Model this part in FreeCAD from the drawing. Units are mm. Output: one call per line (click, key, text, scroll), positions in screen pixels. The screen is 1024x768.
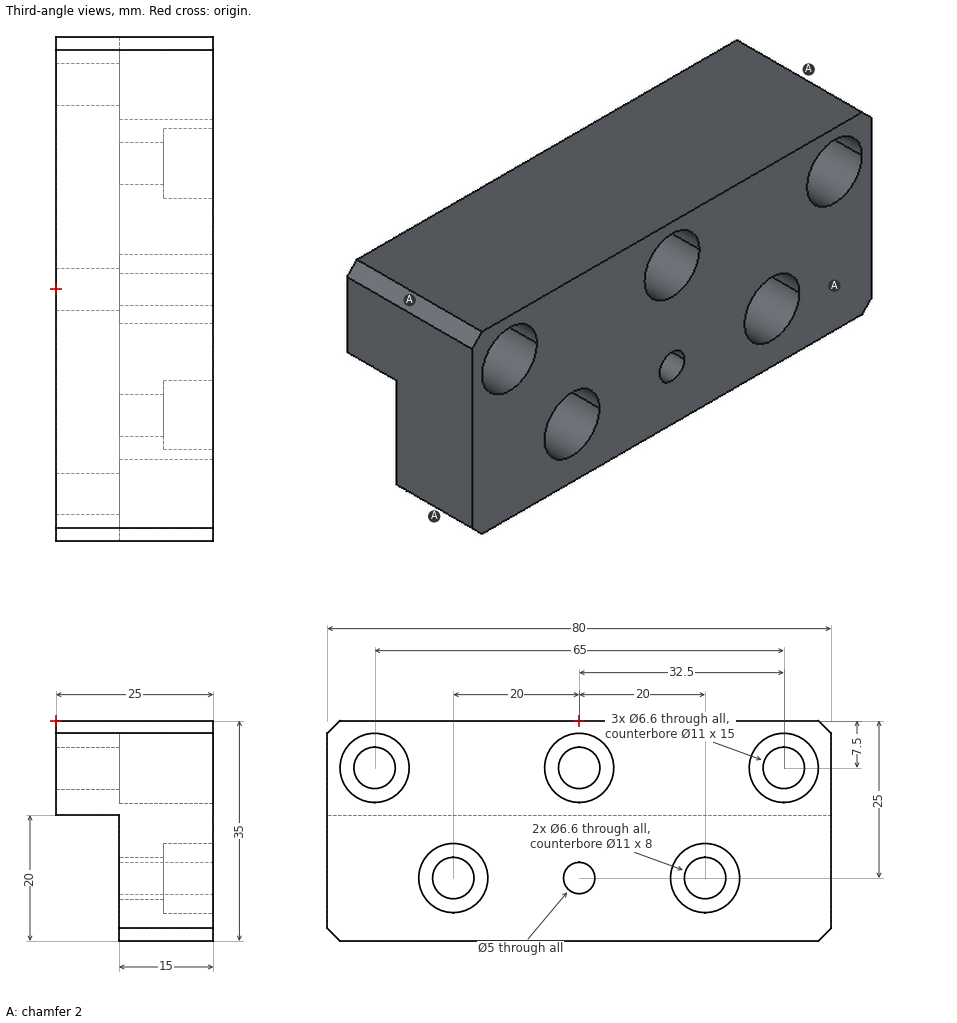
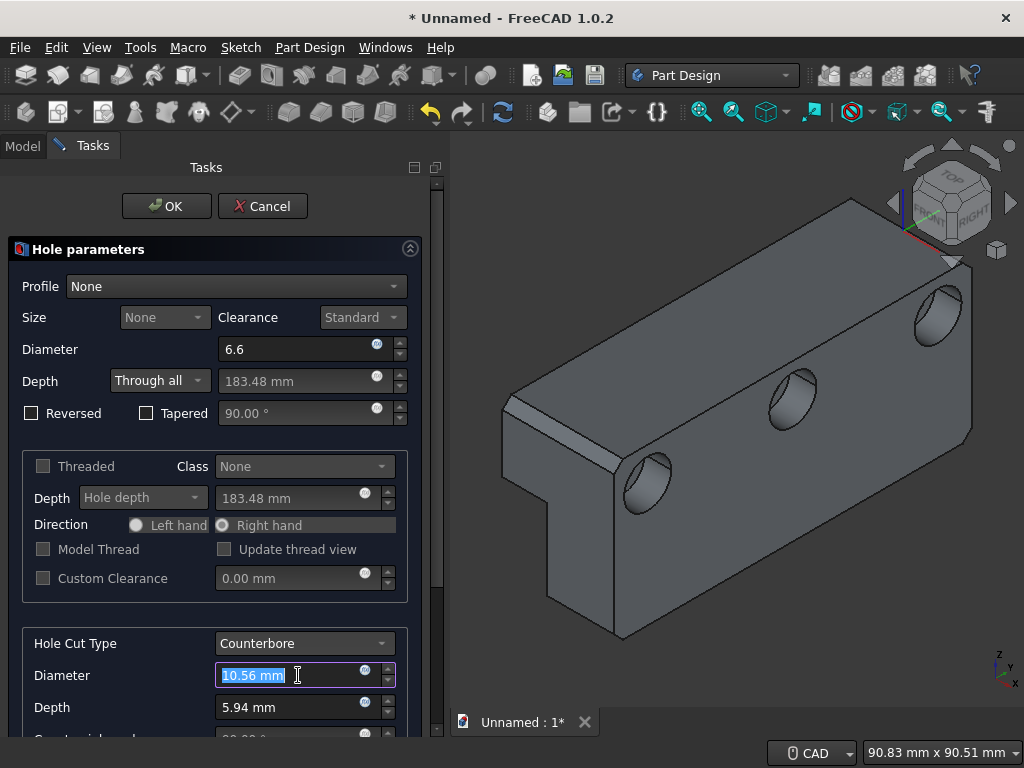
text(11)
key(Tab)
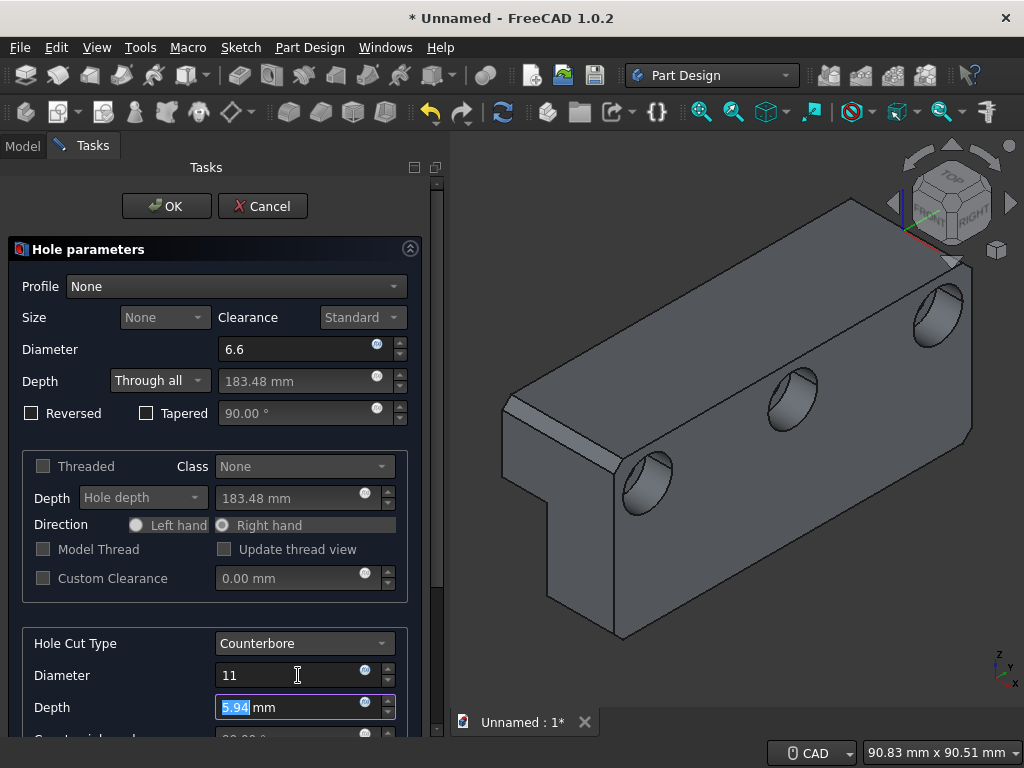
text(15)
key(Tab)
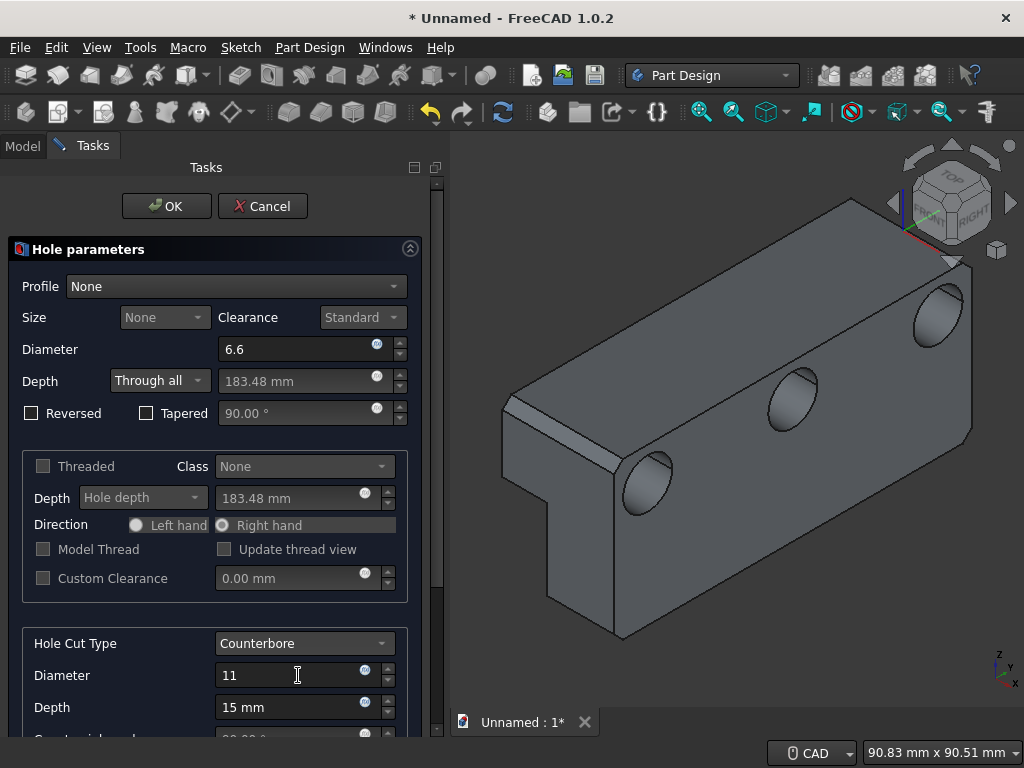
click(167, 206)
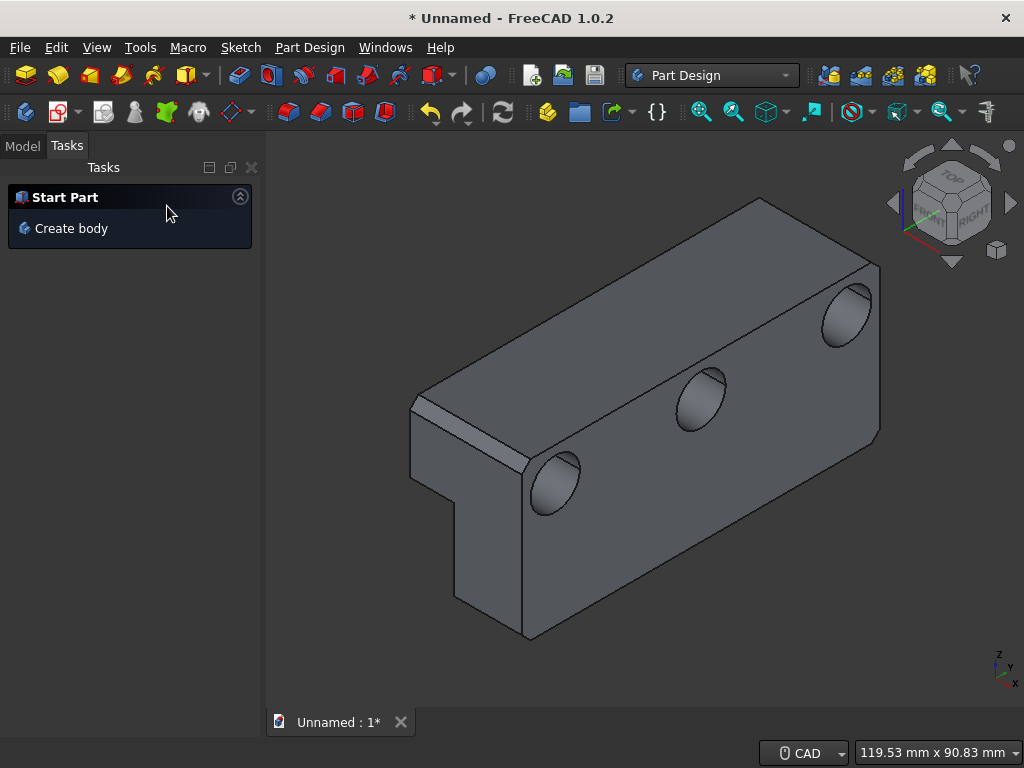
click(752, 447)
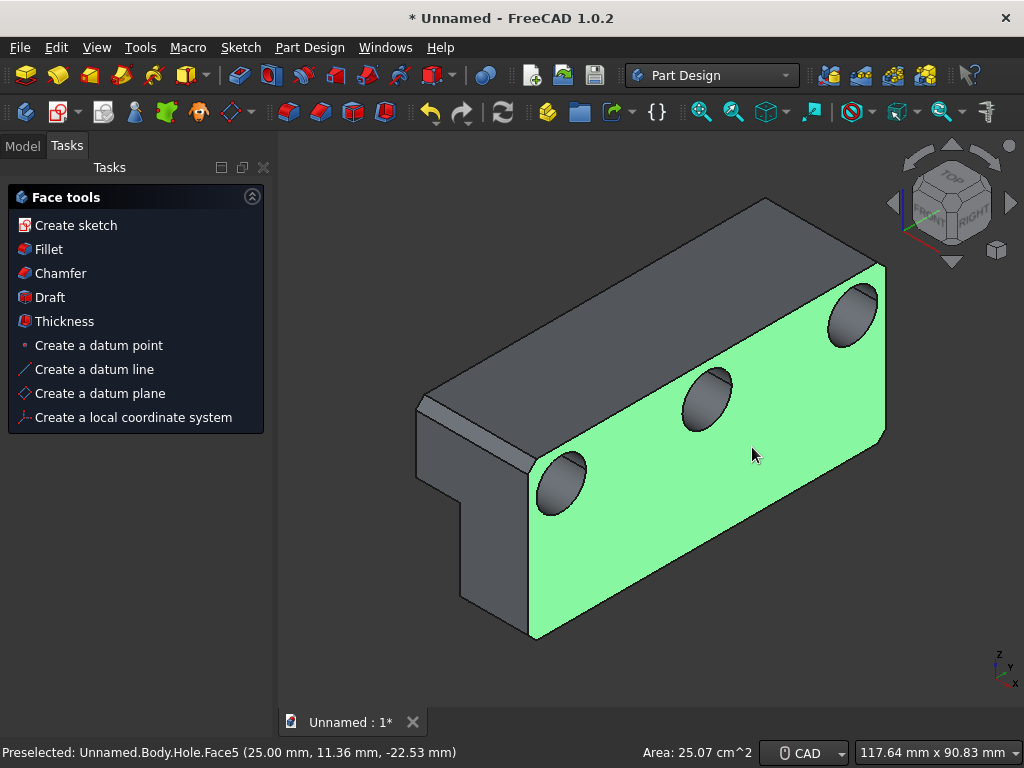
click(58, 112)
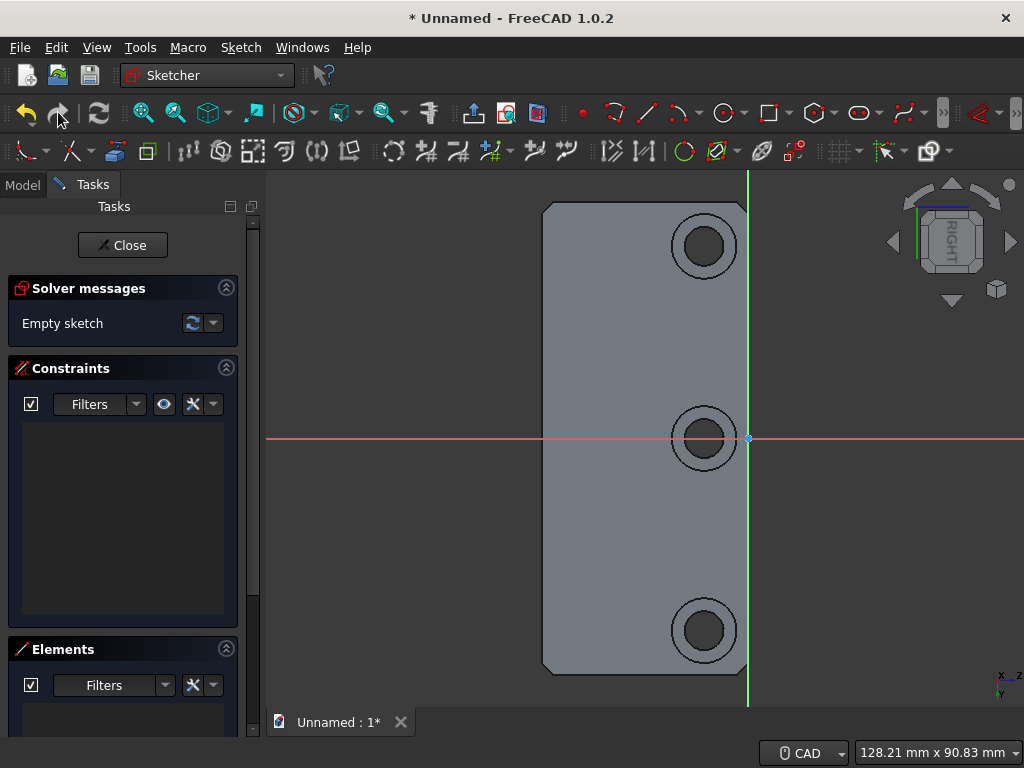
scroll(603, 438, up, 12)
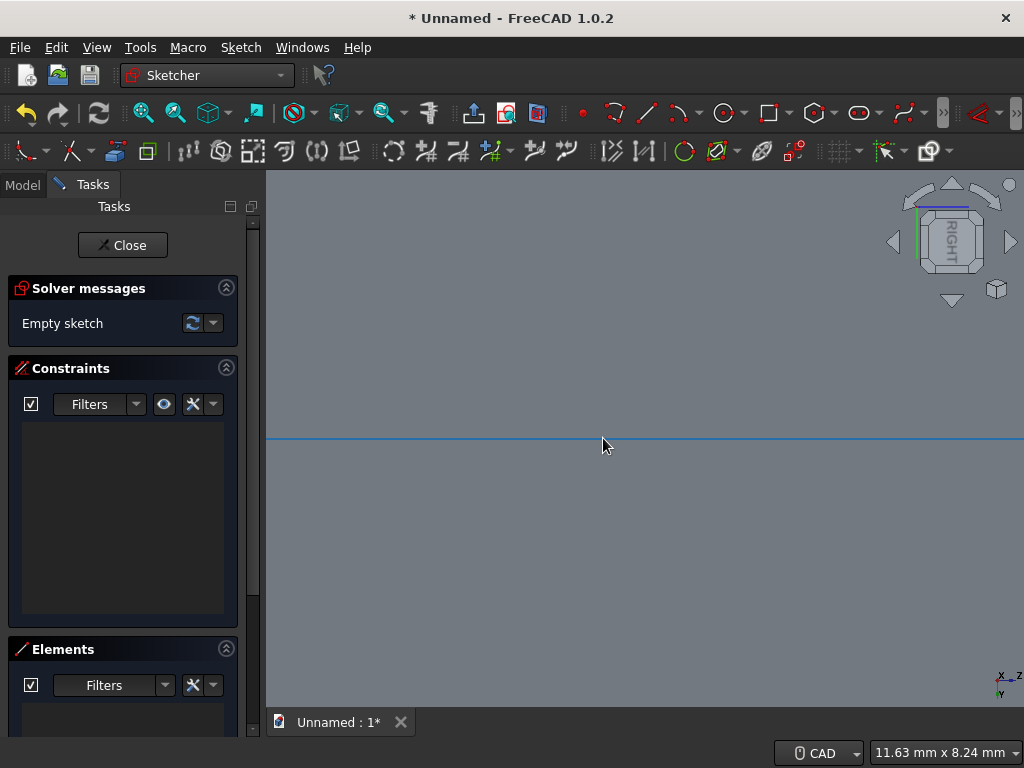
click(724, 114)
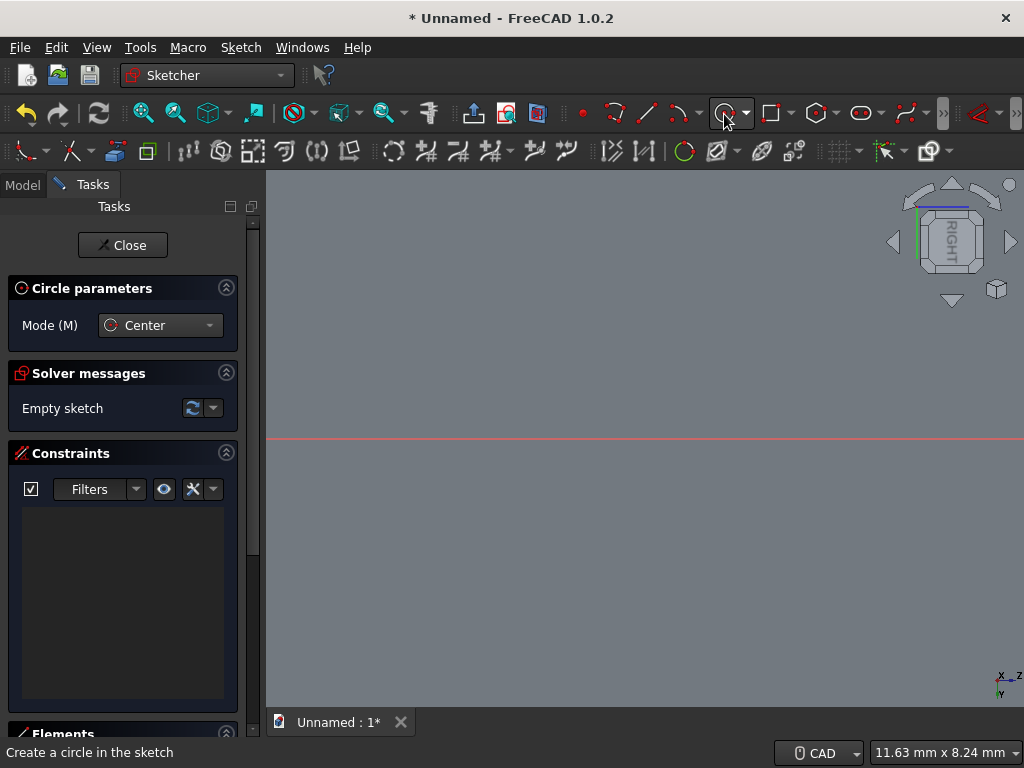
click(573, 438)
click(688, 323)
key(Escape)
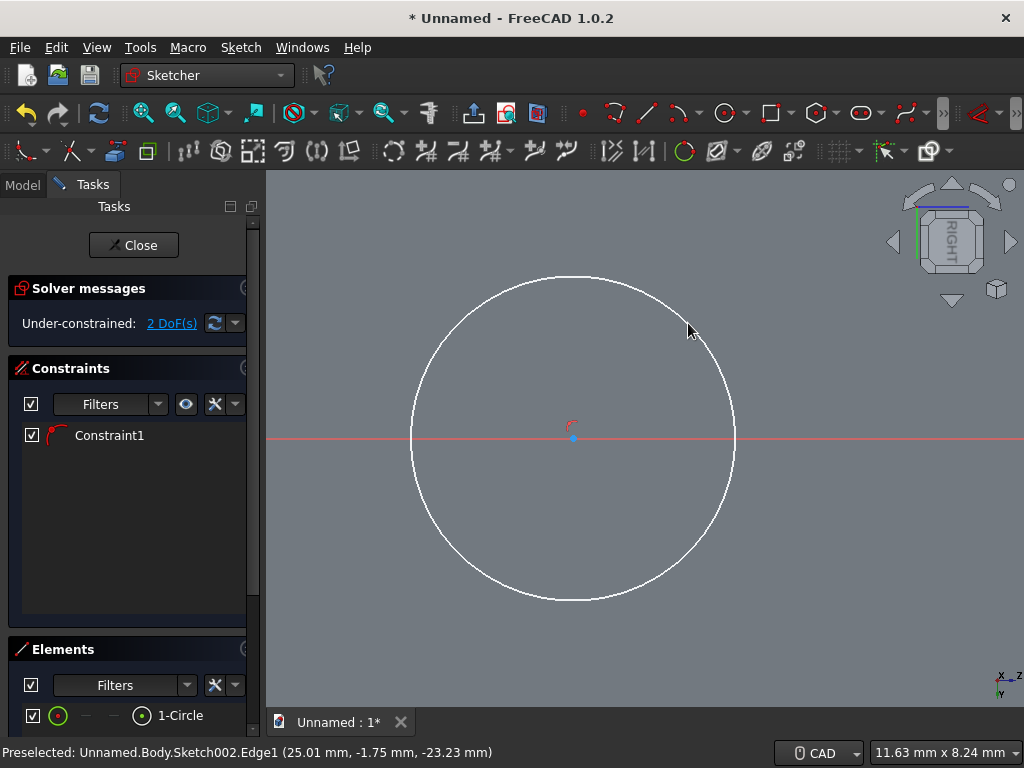
click(978, 114)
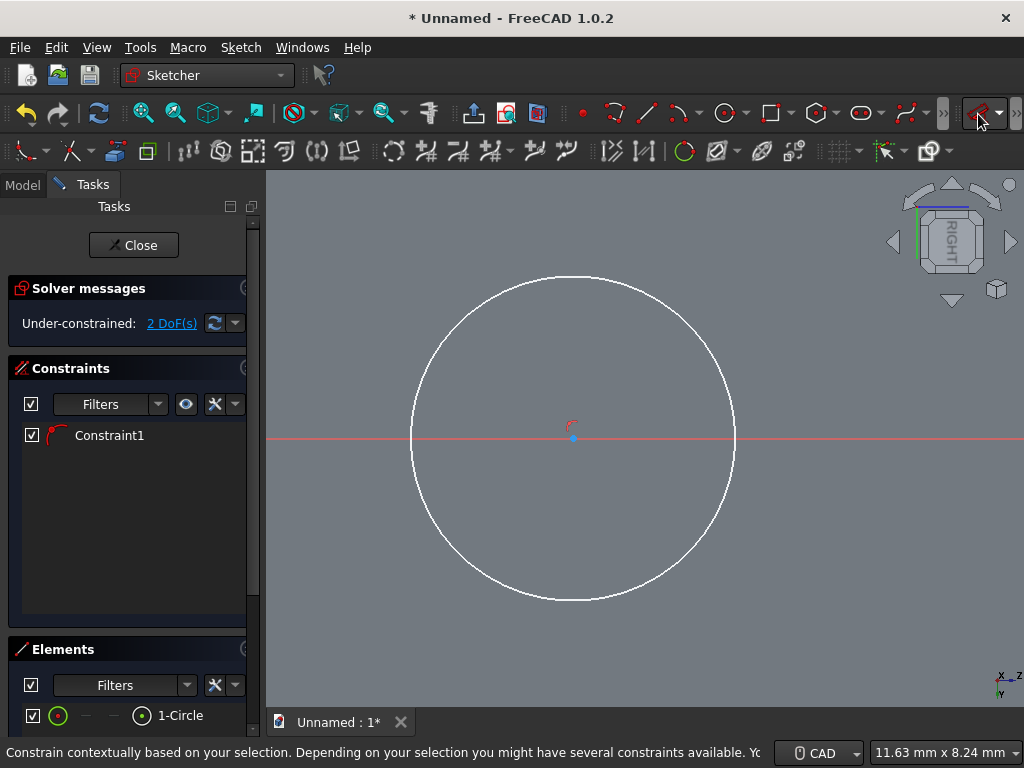
click(687, 323)
click(709, 300)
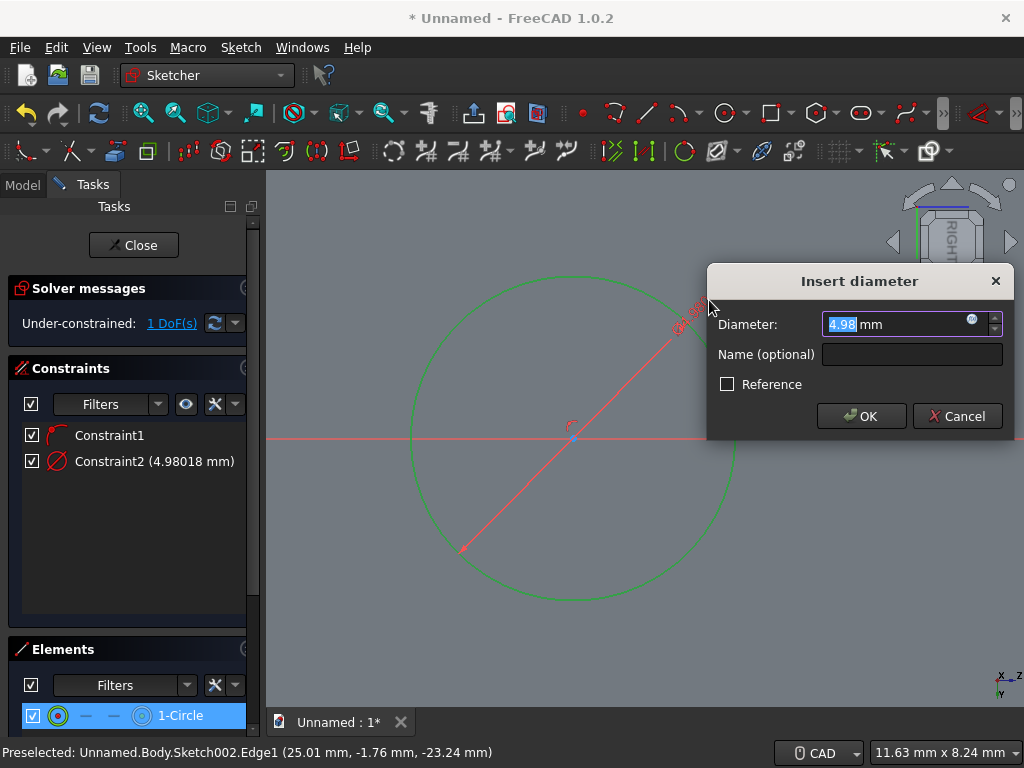
text(5)
key(Return)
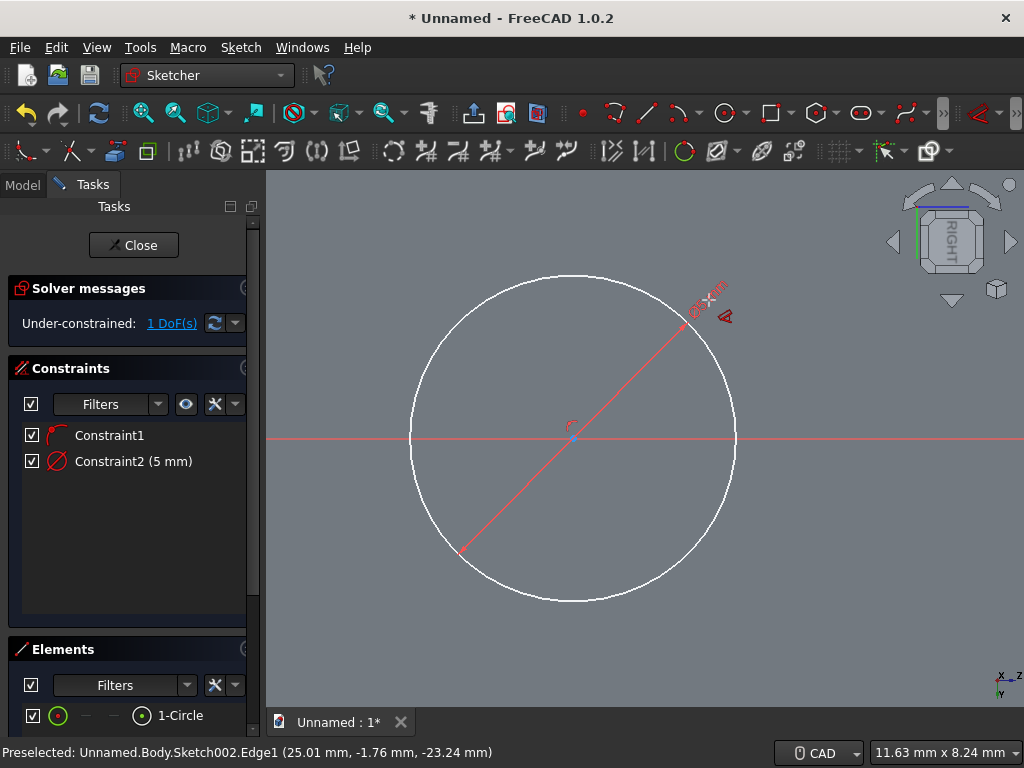
click(573, 438)
click(716, 472)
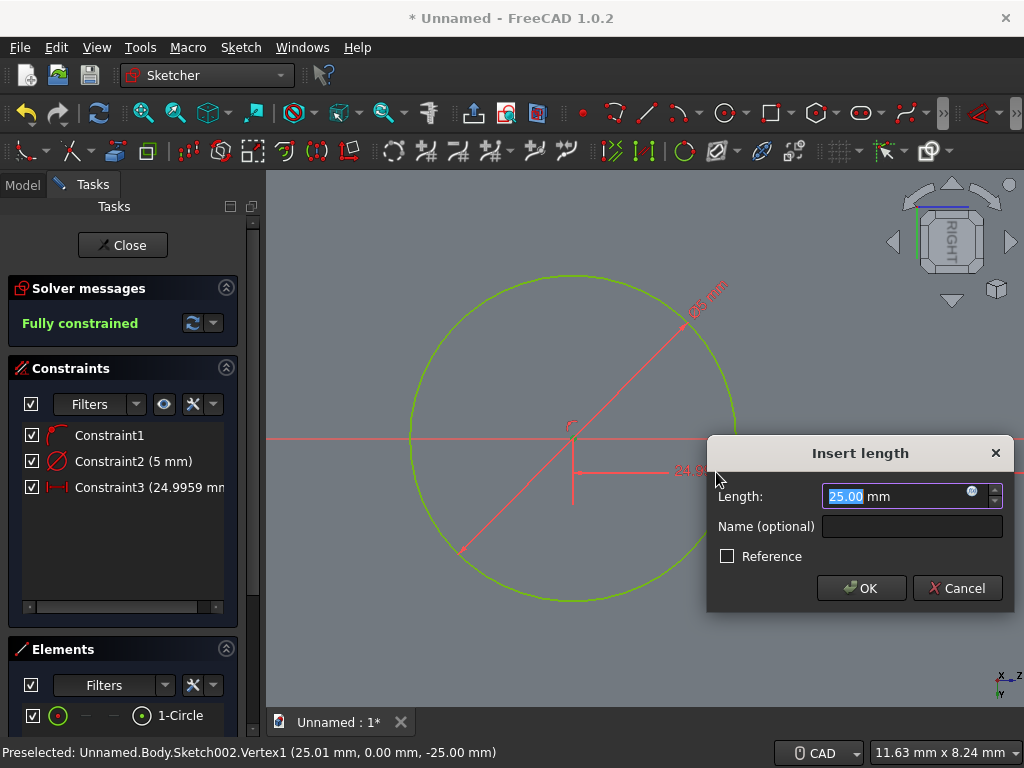
text(25)
key(Return)
key(Escape)